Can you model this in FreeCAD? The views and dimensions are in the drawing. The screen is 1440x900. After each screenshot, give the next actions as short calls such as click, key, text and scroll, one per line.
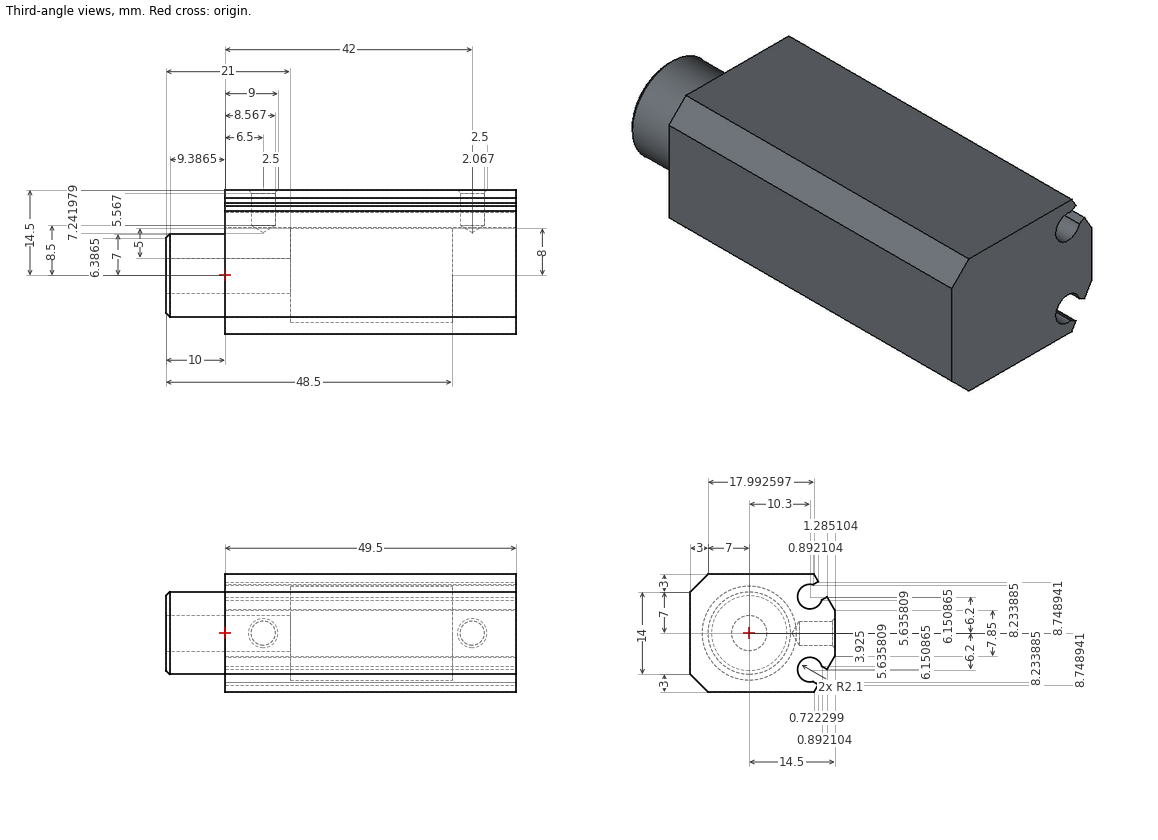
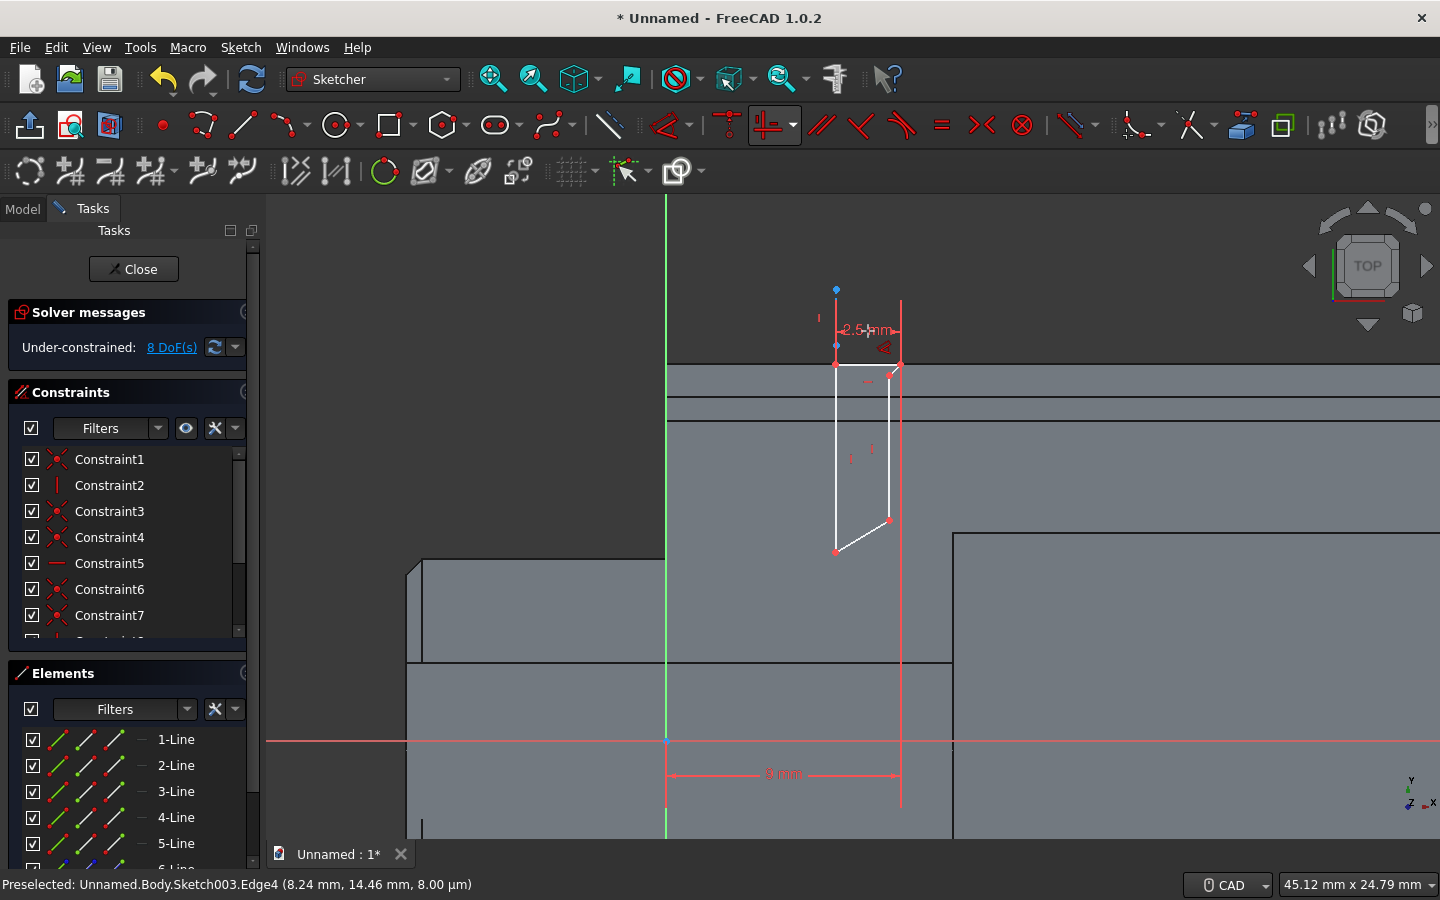
click(889, 521)
click(632, 631)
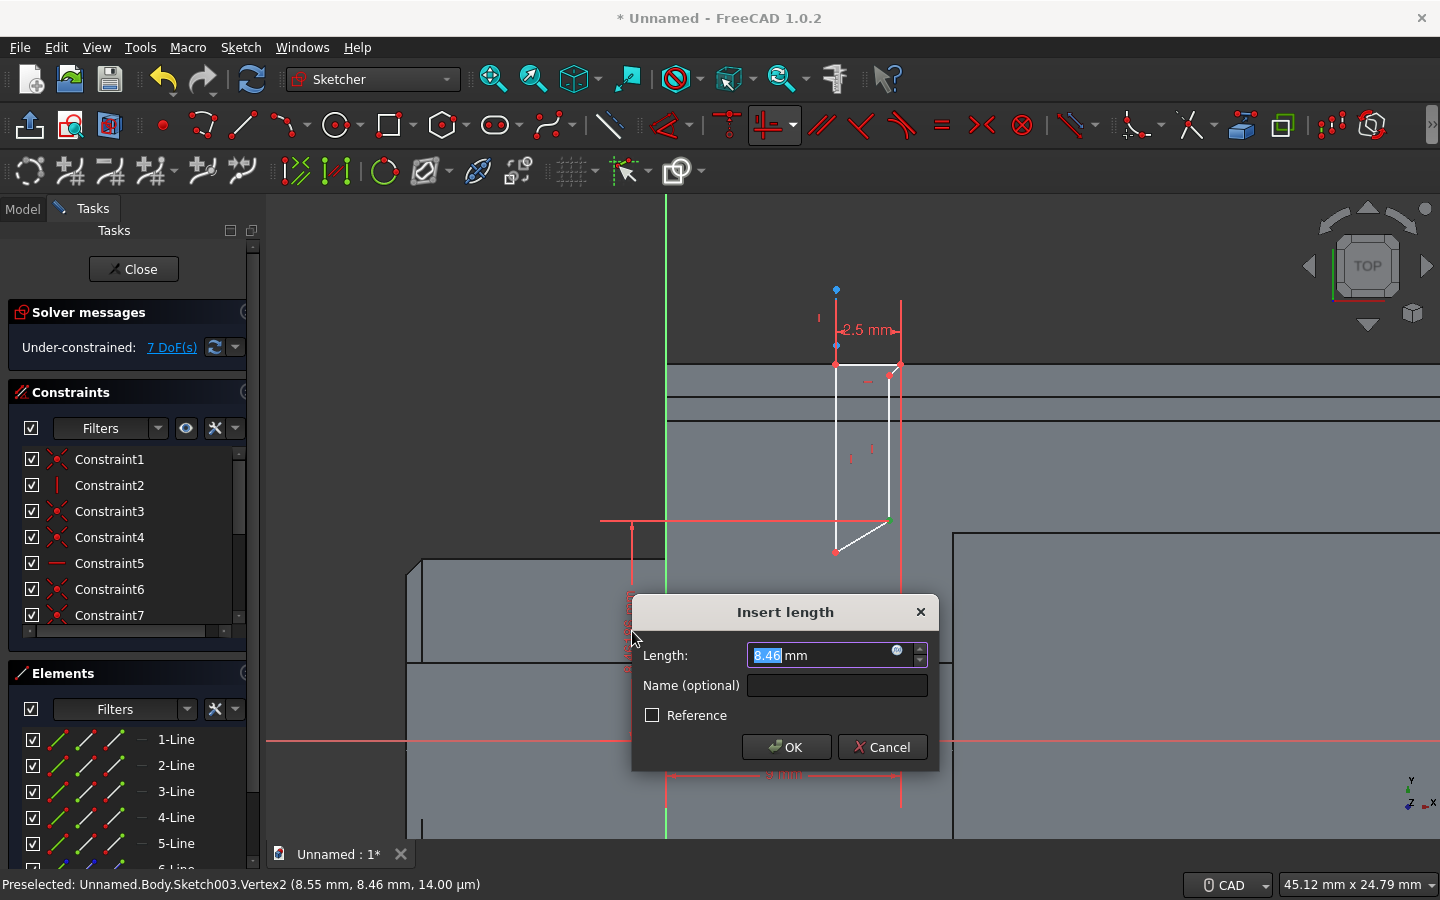
text(8.5)
key(Return)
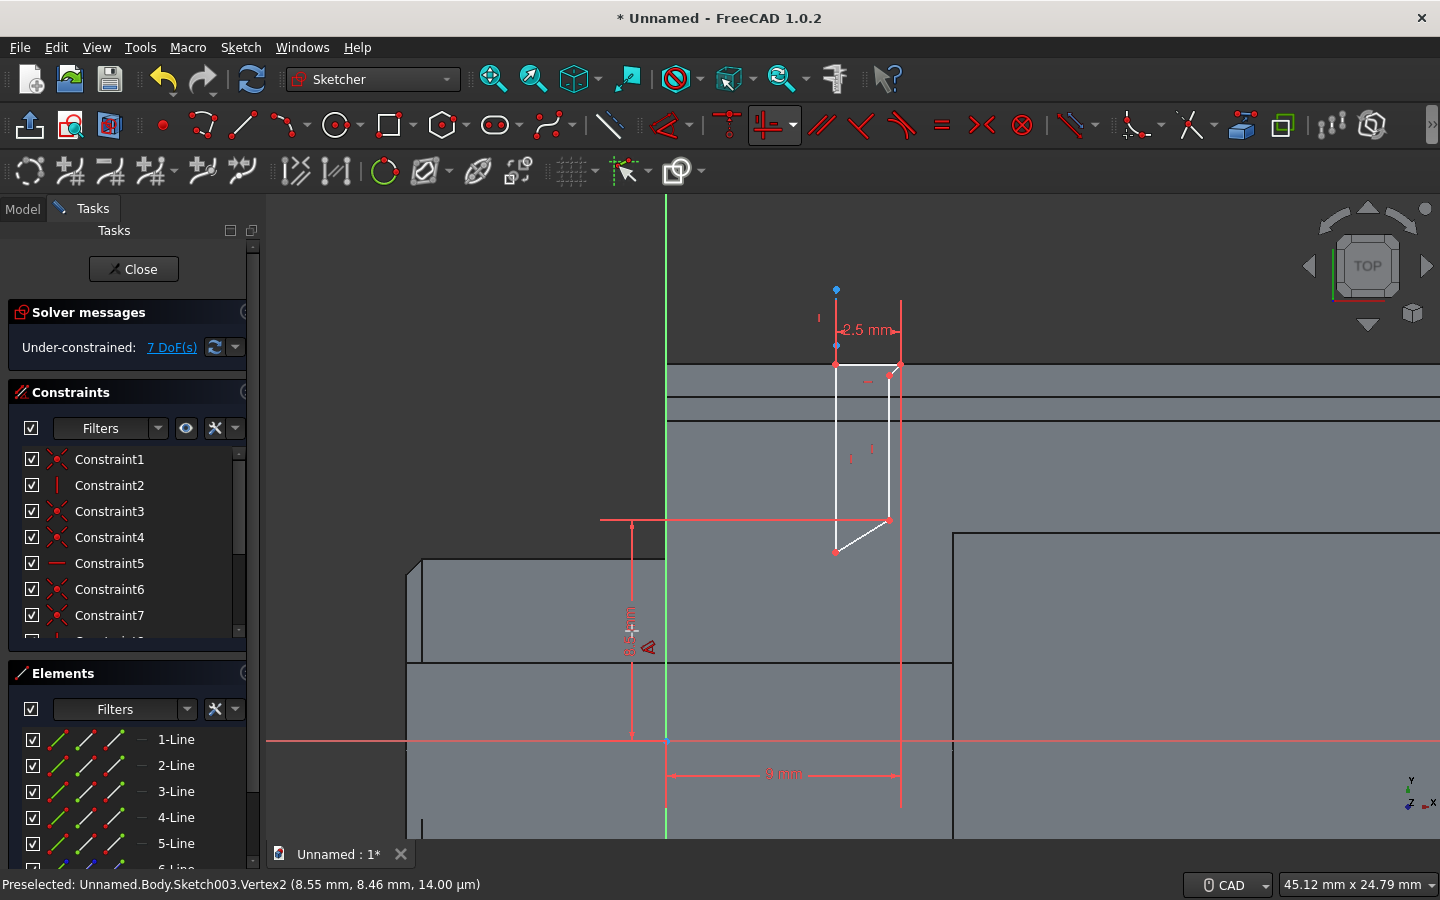
click(836, 346)
click(712, 775)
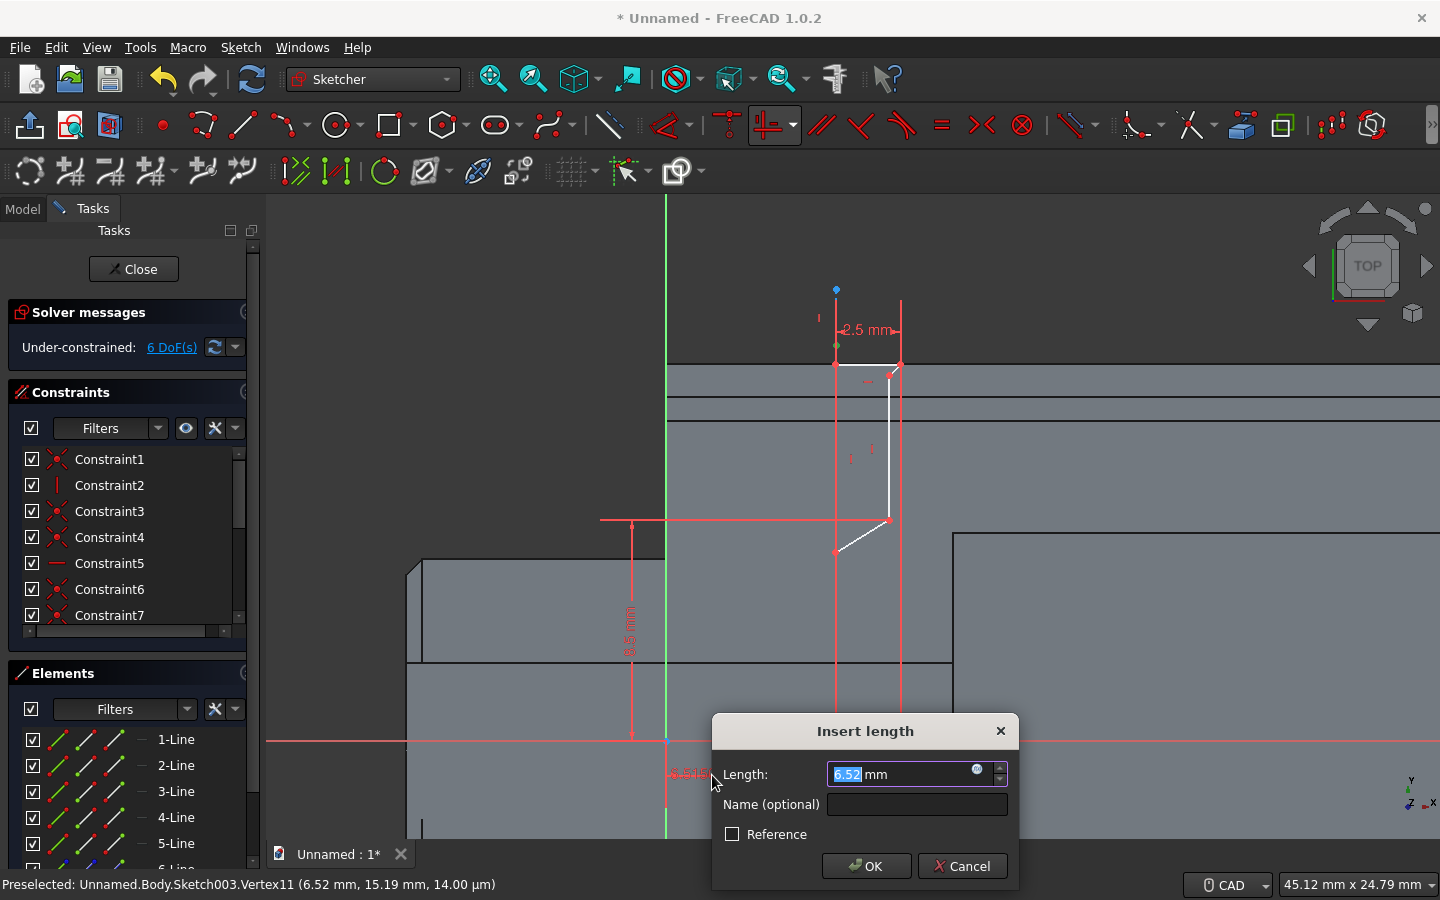
text(6.5)
key(Return)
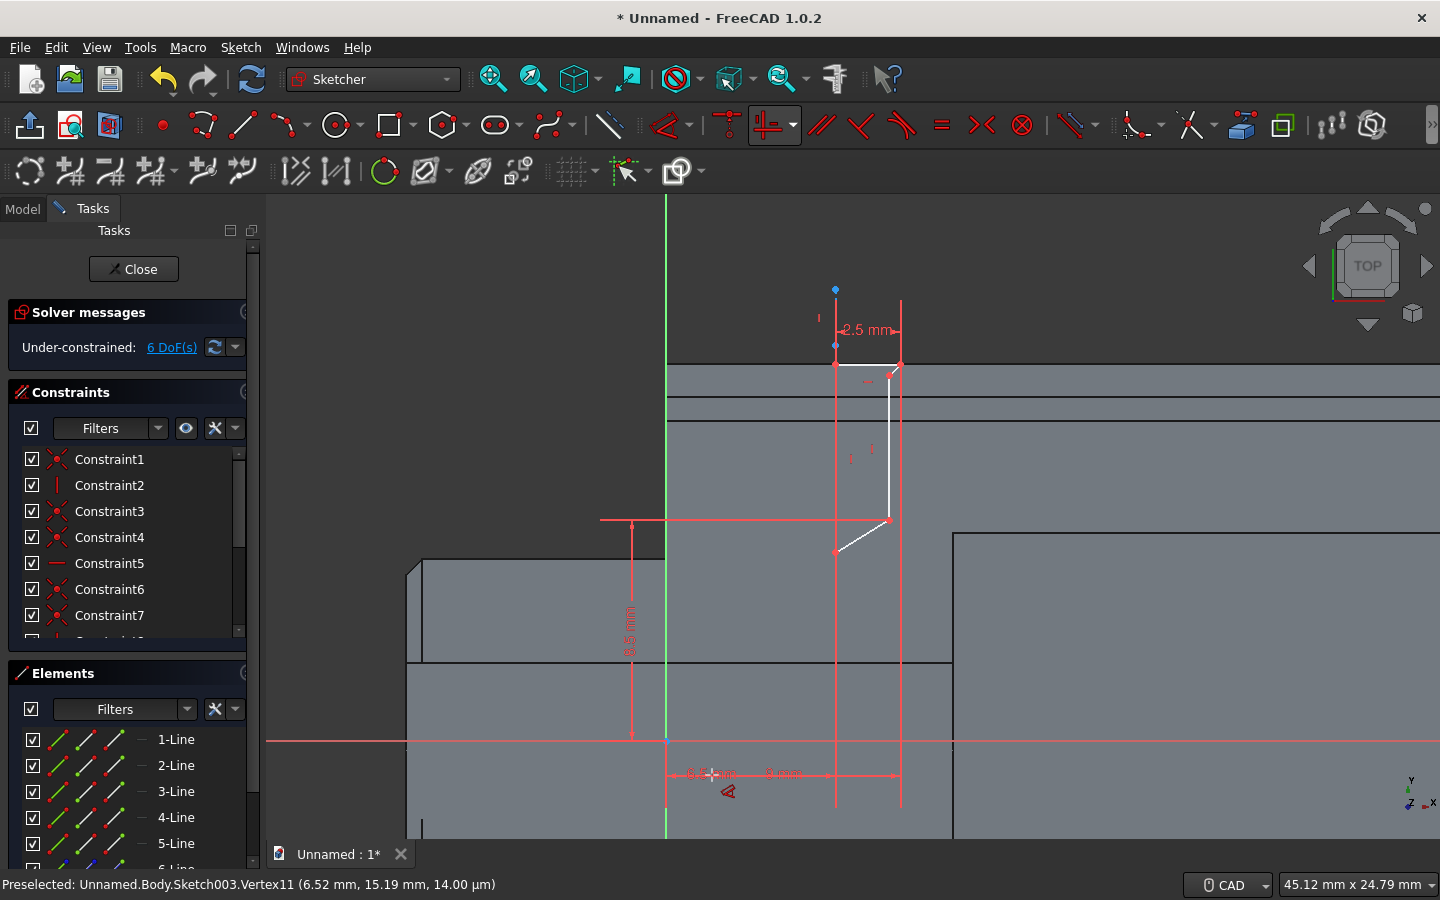
click(889, 477)
click(923, 448)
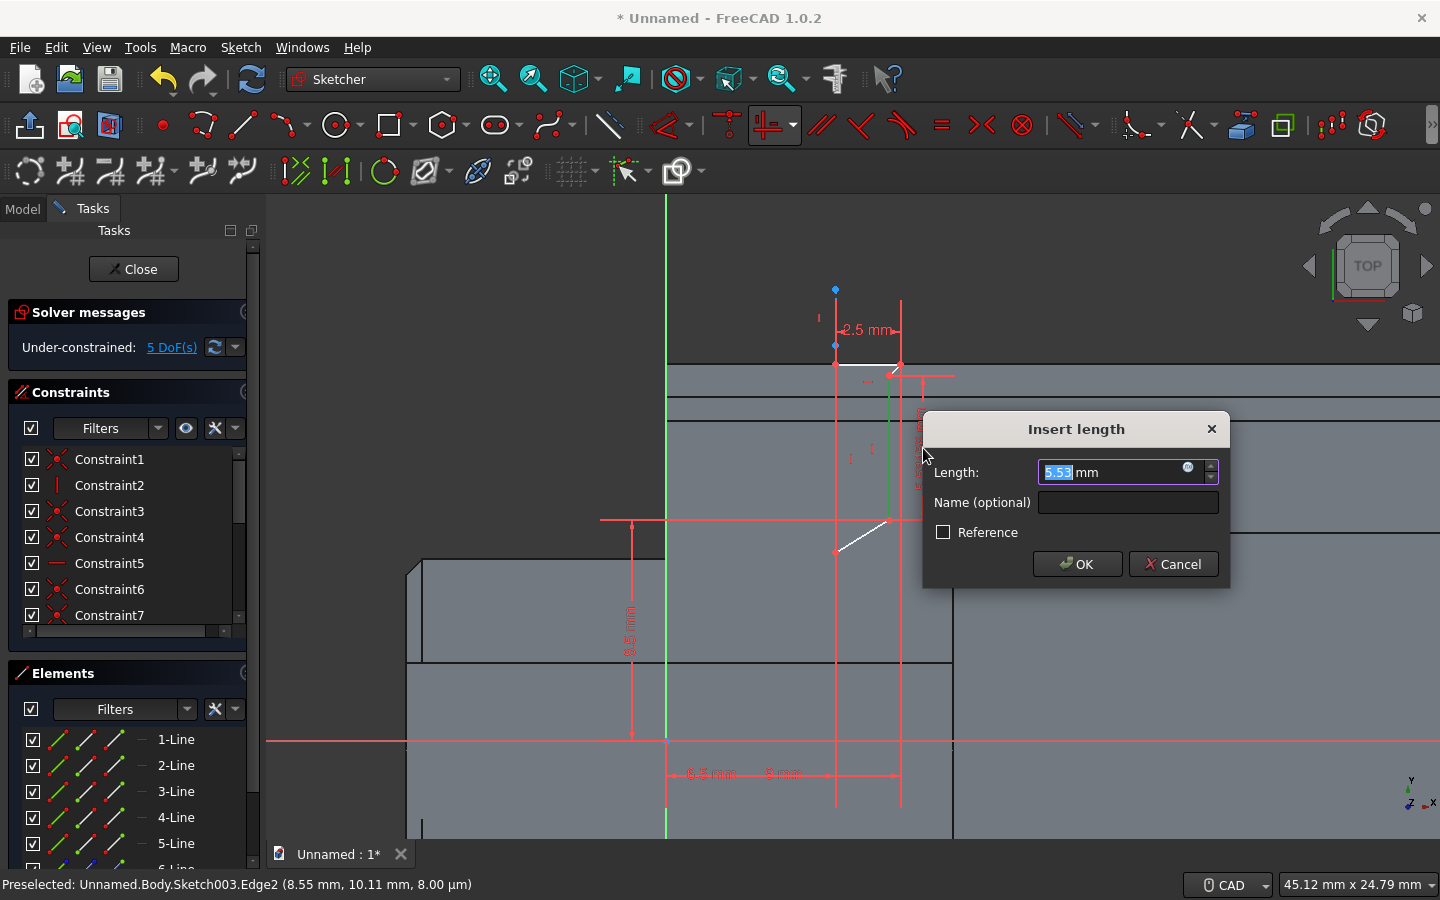
text(5.567)
key(Return)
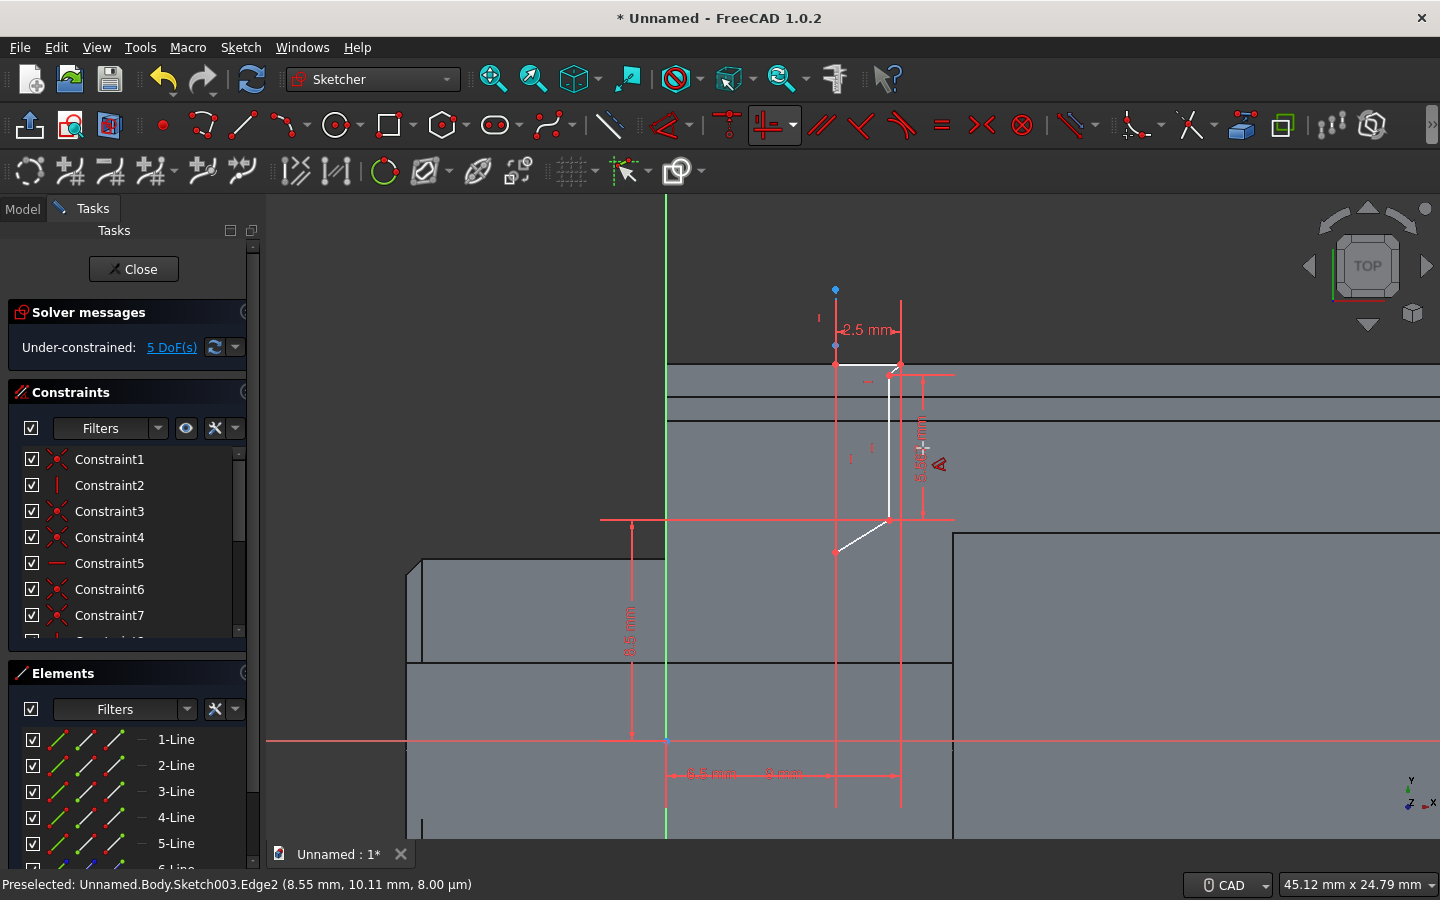
click(901, 365)
click(935, 553)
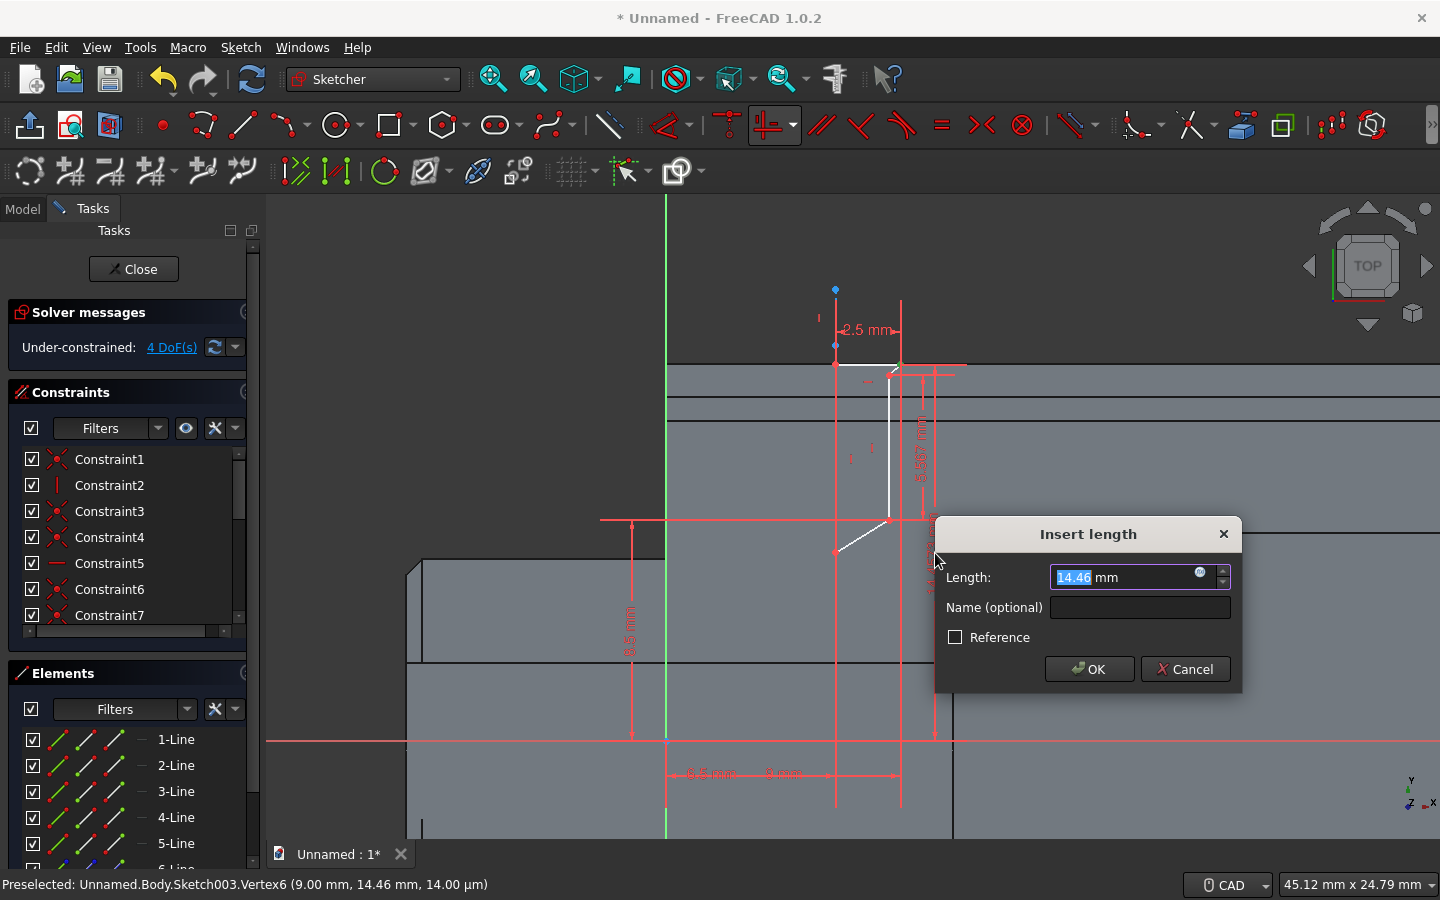
text(14.5)
key(Return)